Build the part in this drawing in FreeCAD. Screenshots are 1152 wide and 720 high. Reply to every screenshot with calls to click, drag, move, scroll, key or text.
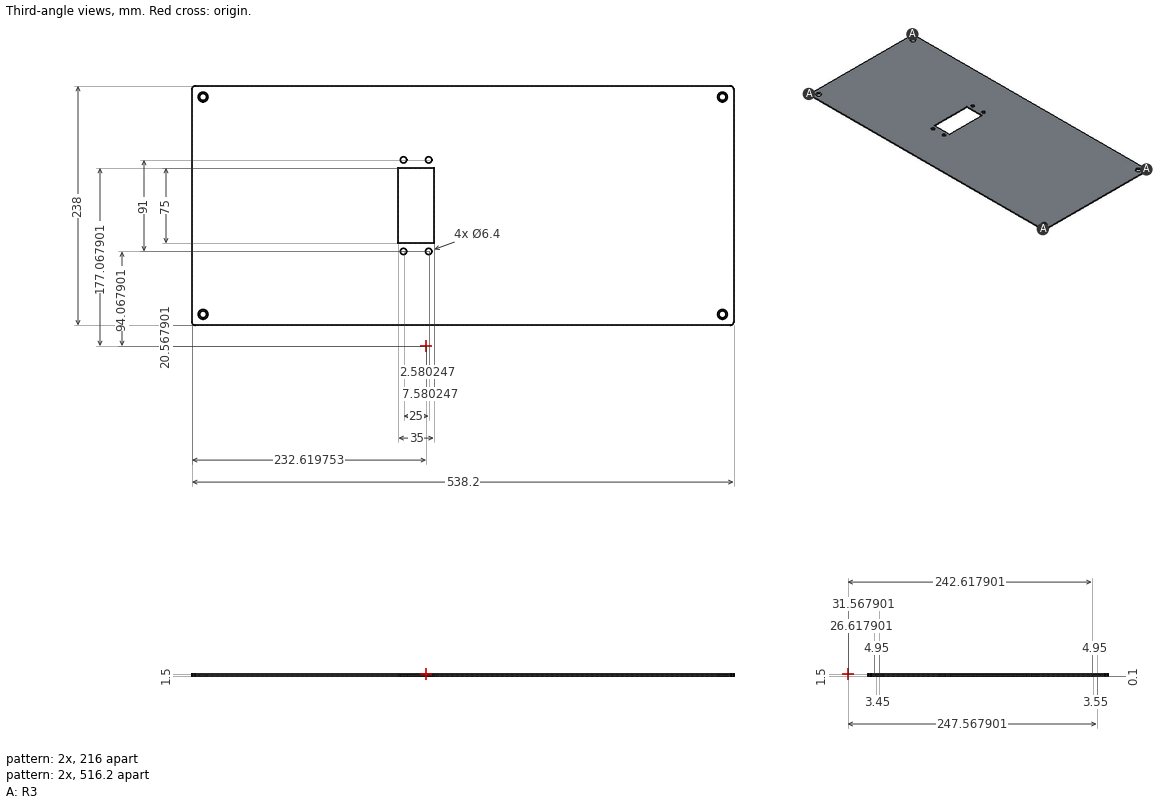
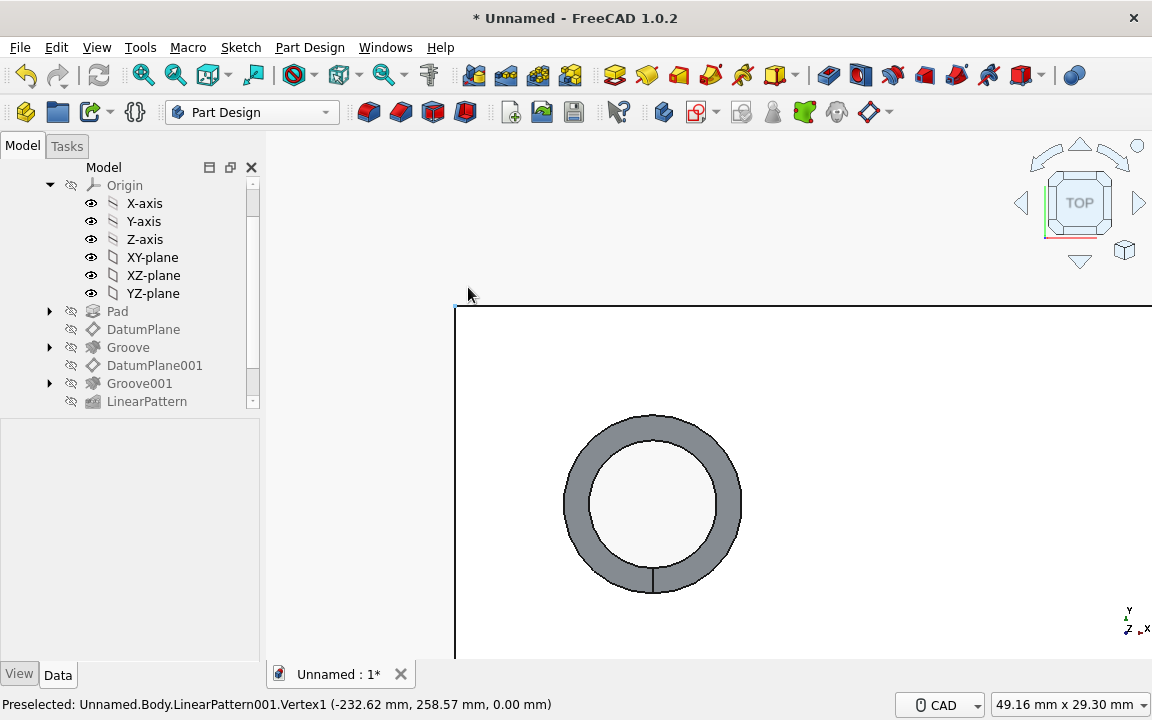
click(144, 76)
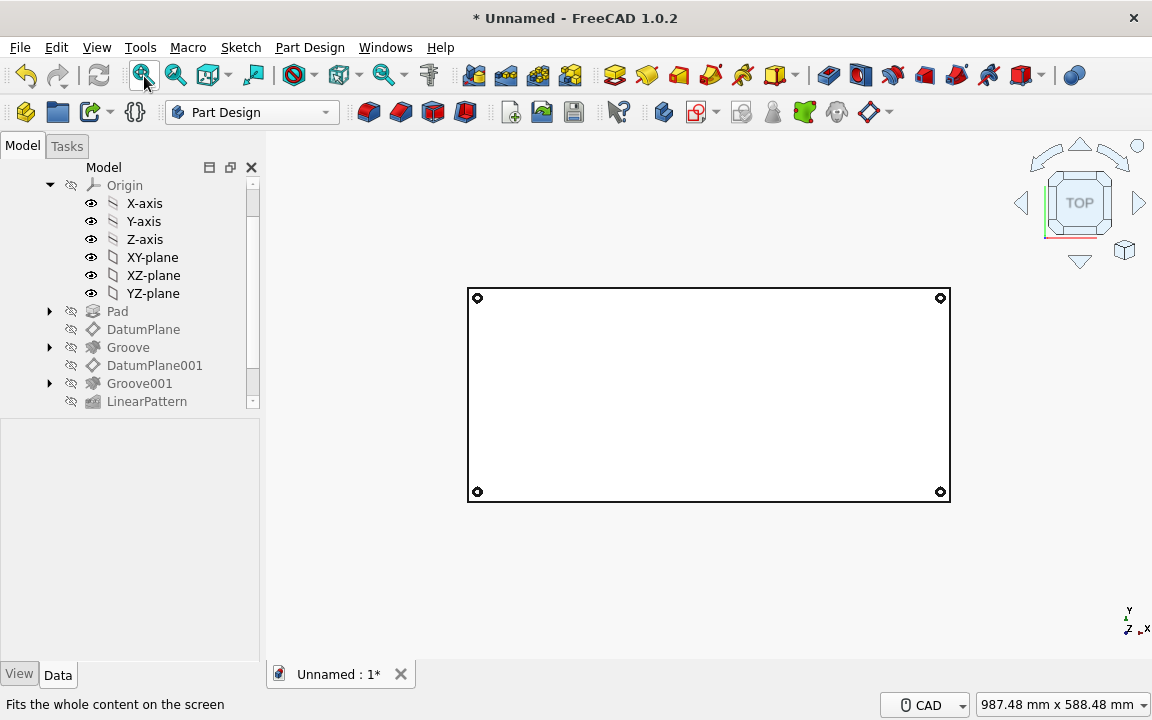
key(1)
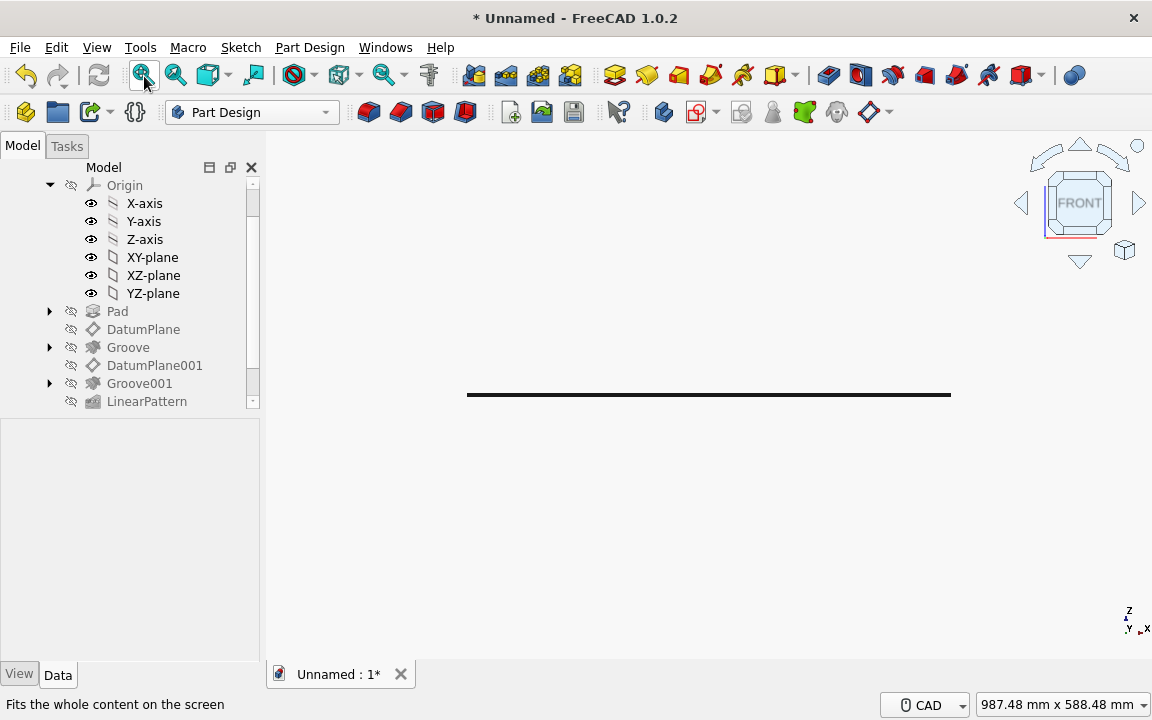
scroll(468, 394, up, 15)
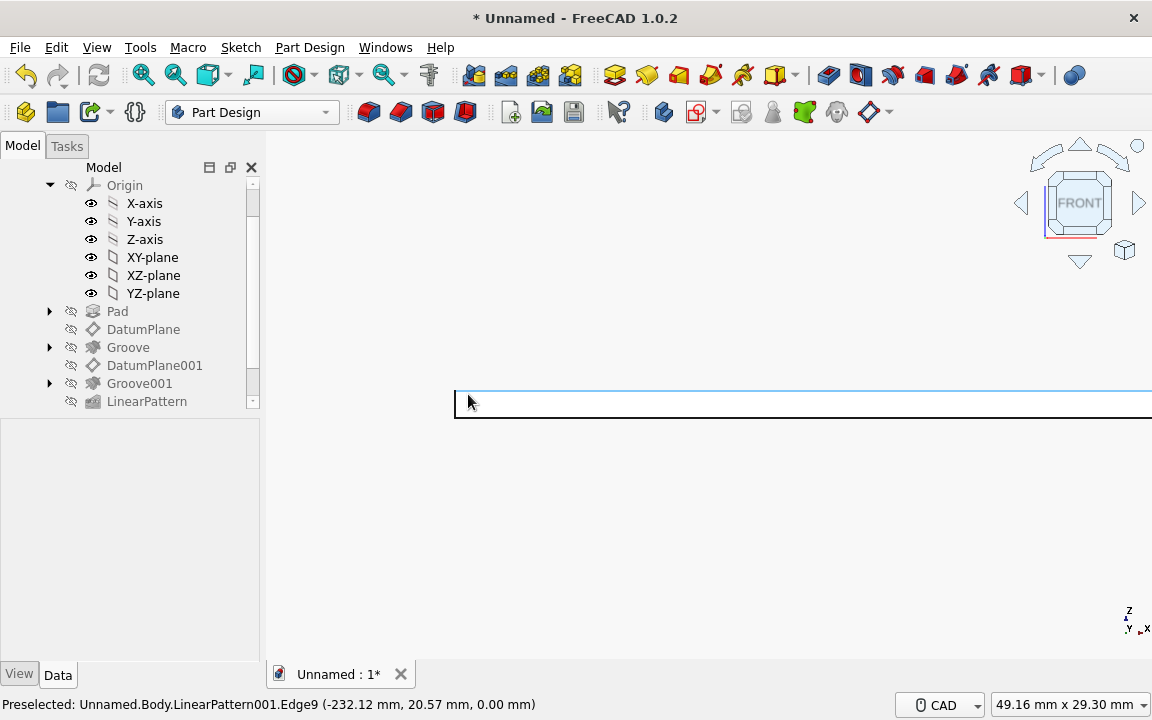
click(455, 404)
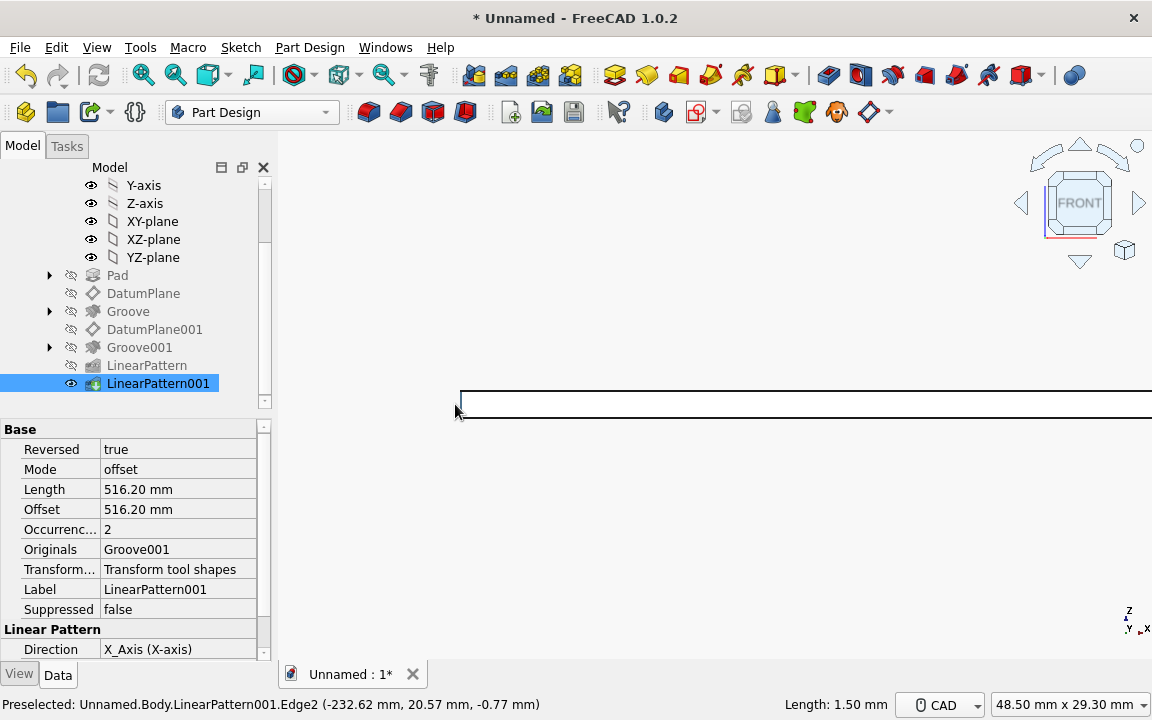
click(144, 76)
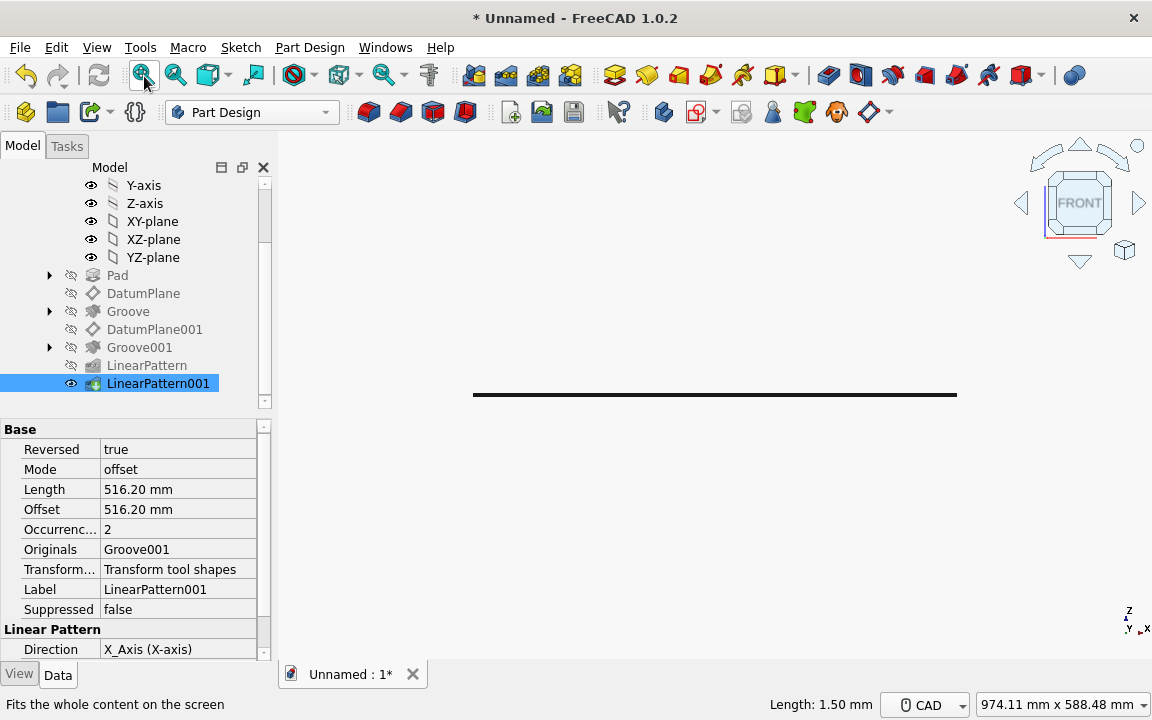
key(3)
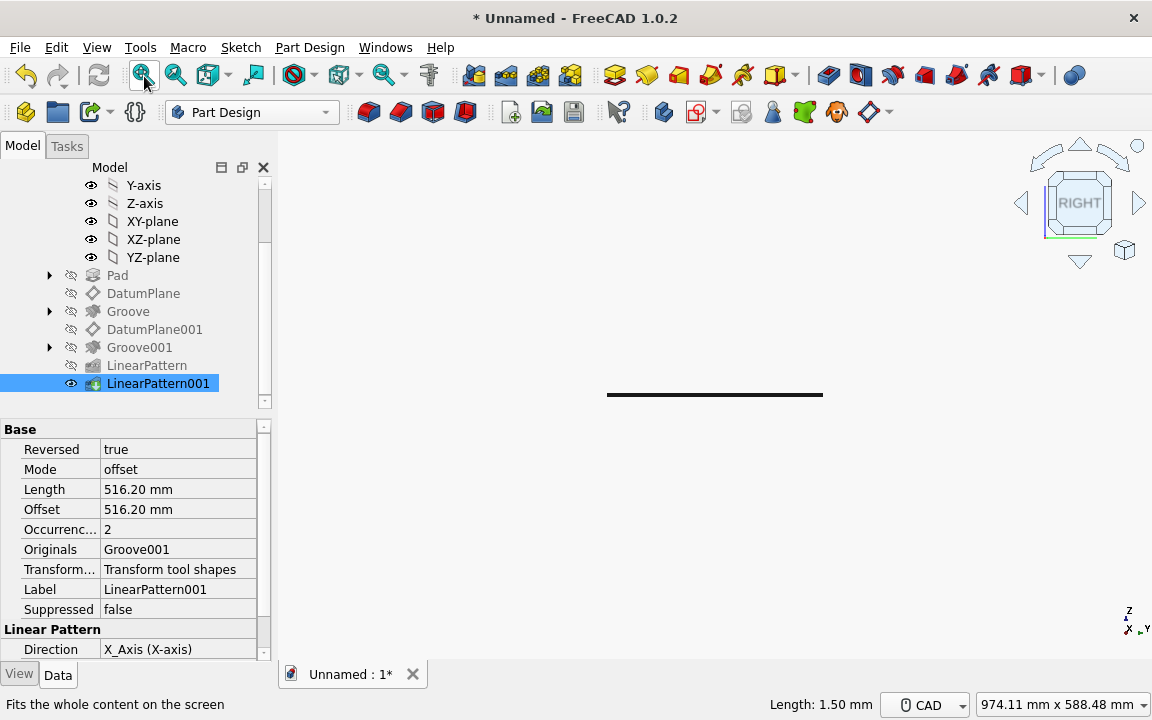
click(144, 76)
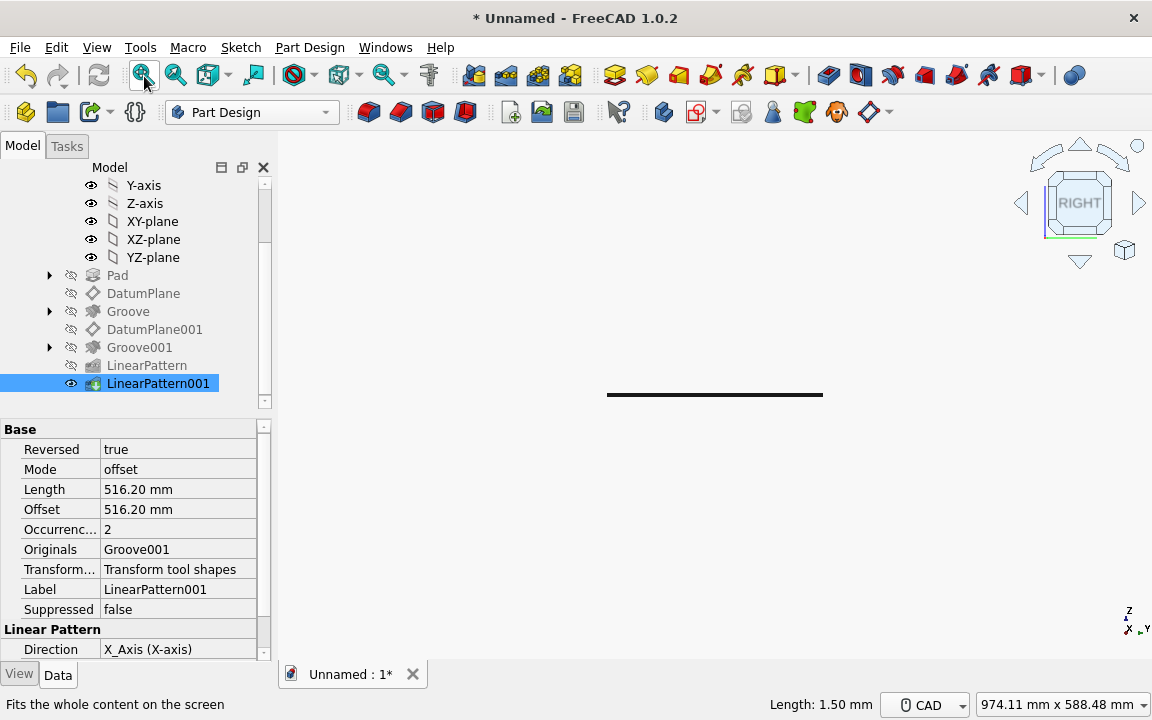
scroll(822, 394, up, 15)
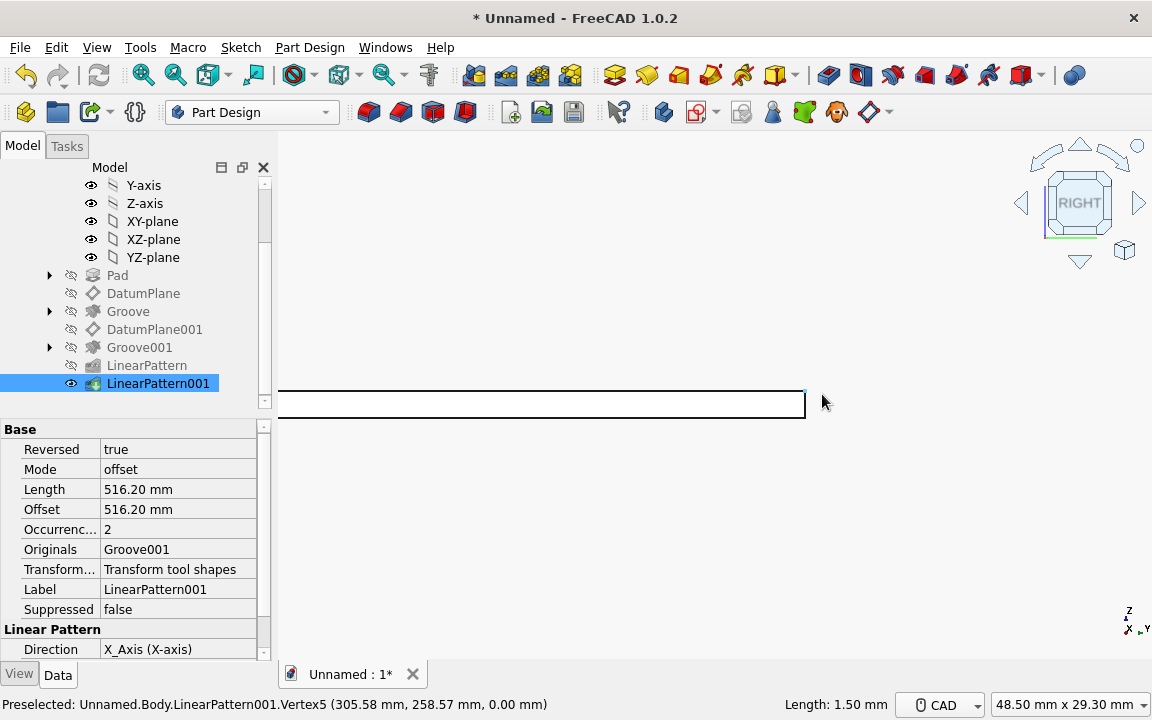
click(805, 404, ctrl)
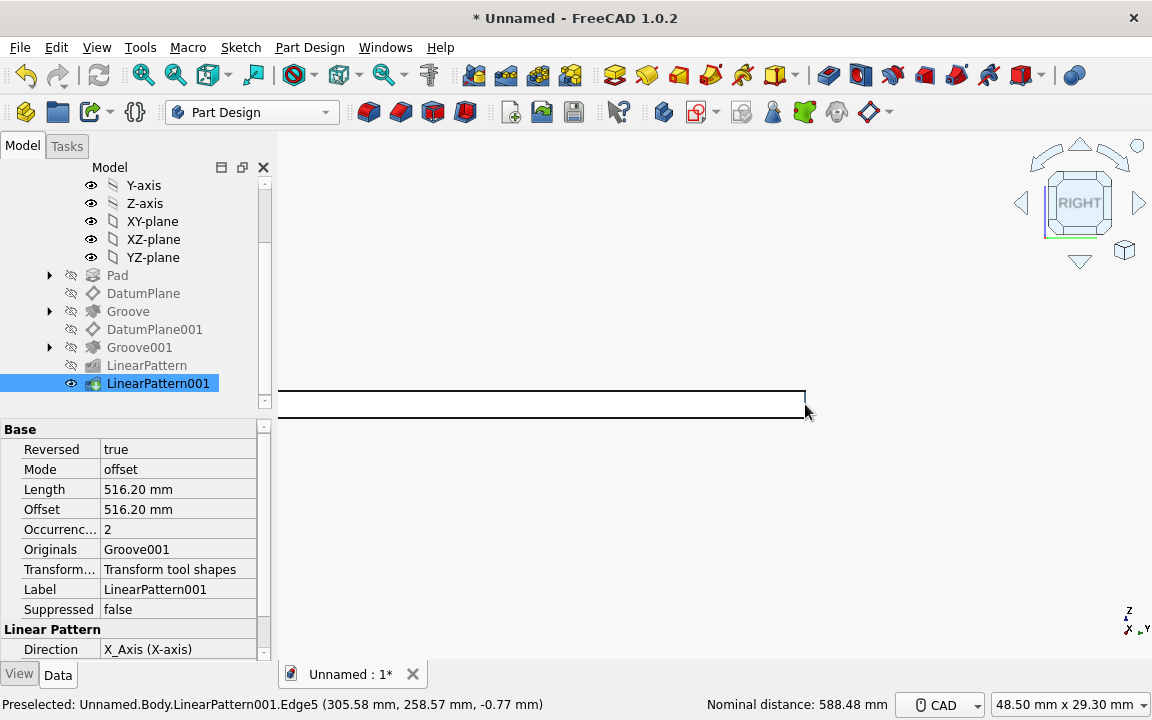
click(144, 76)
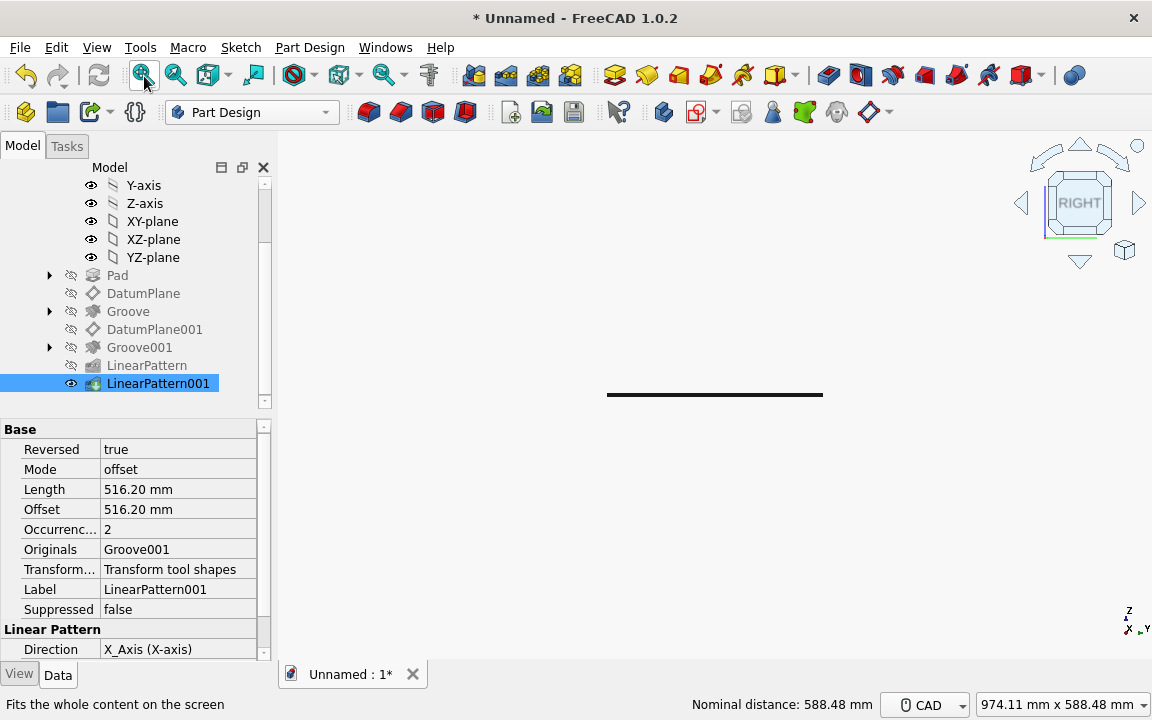
key(5)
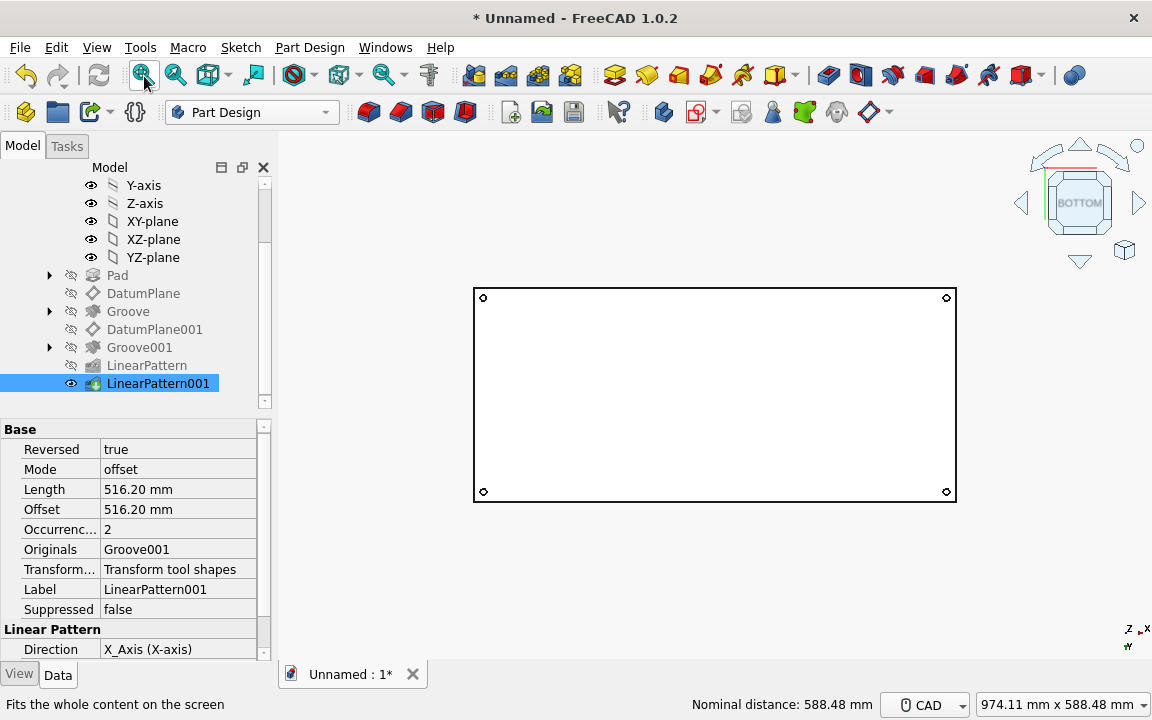
scroll(474, 501, up, 15)